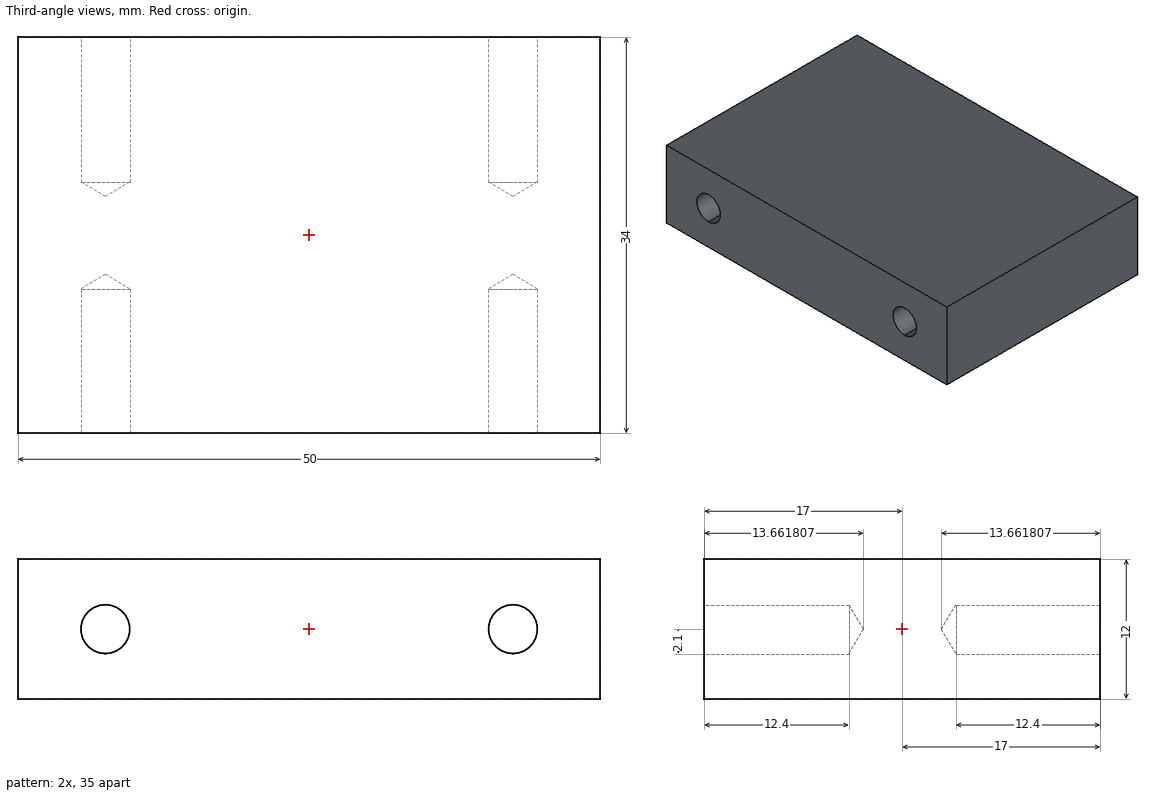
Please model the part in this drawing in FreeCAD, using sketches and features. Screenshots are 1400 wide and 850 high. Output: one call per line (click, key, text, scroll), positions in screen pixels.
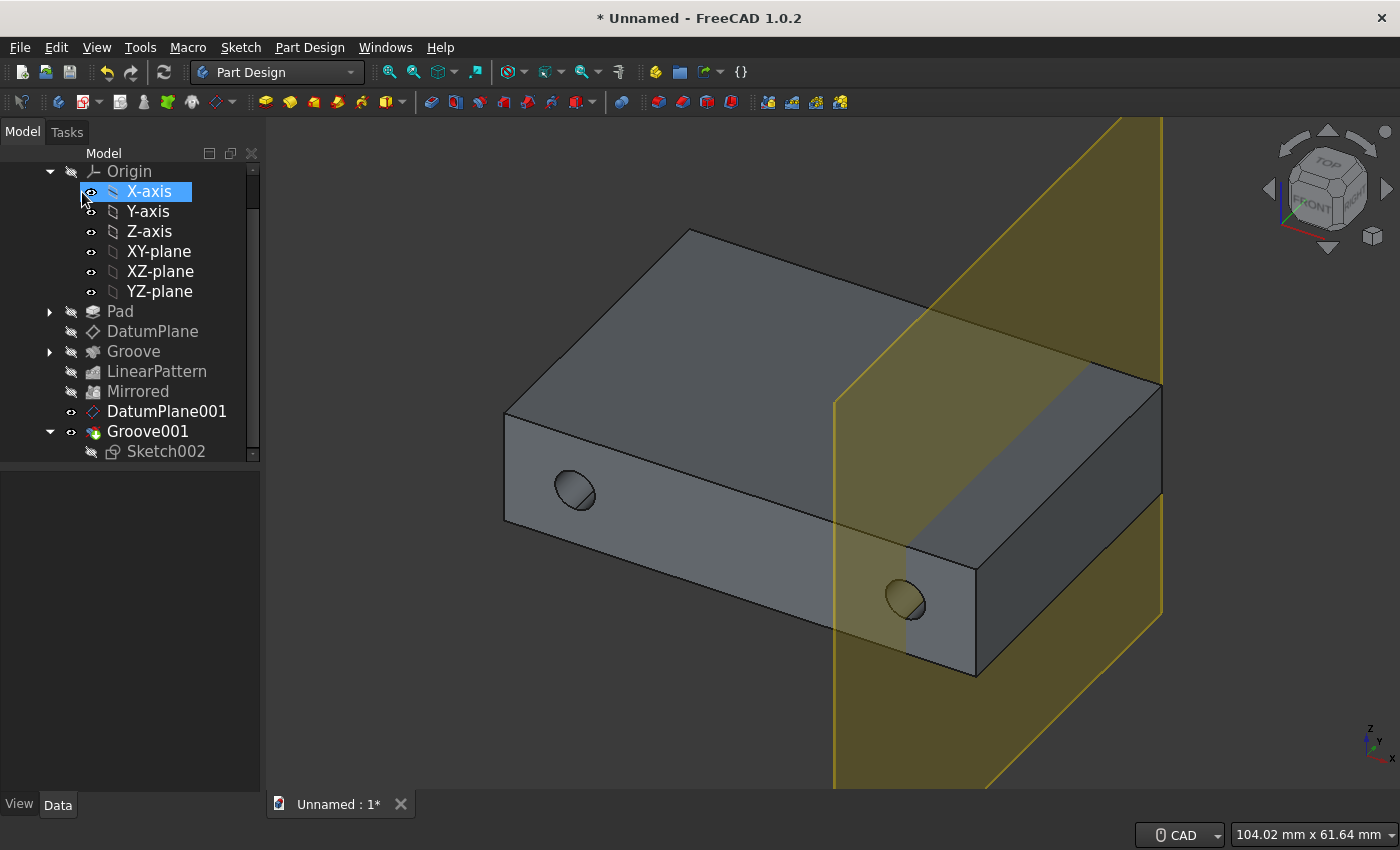
click(116, 412)
key(space)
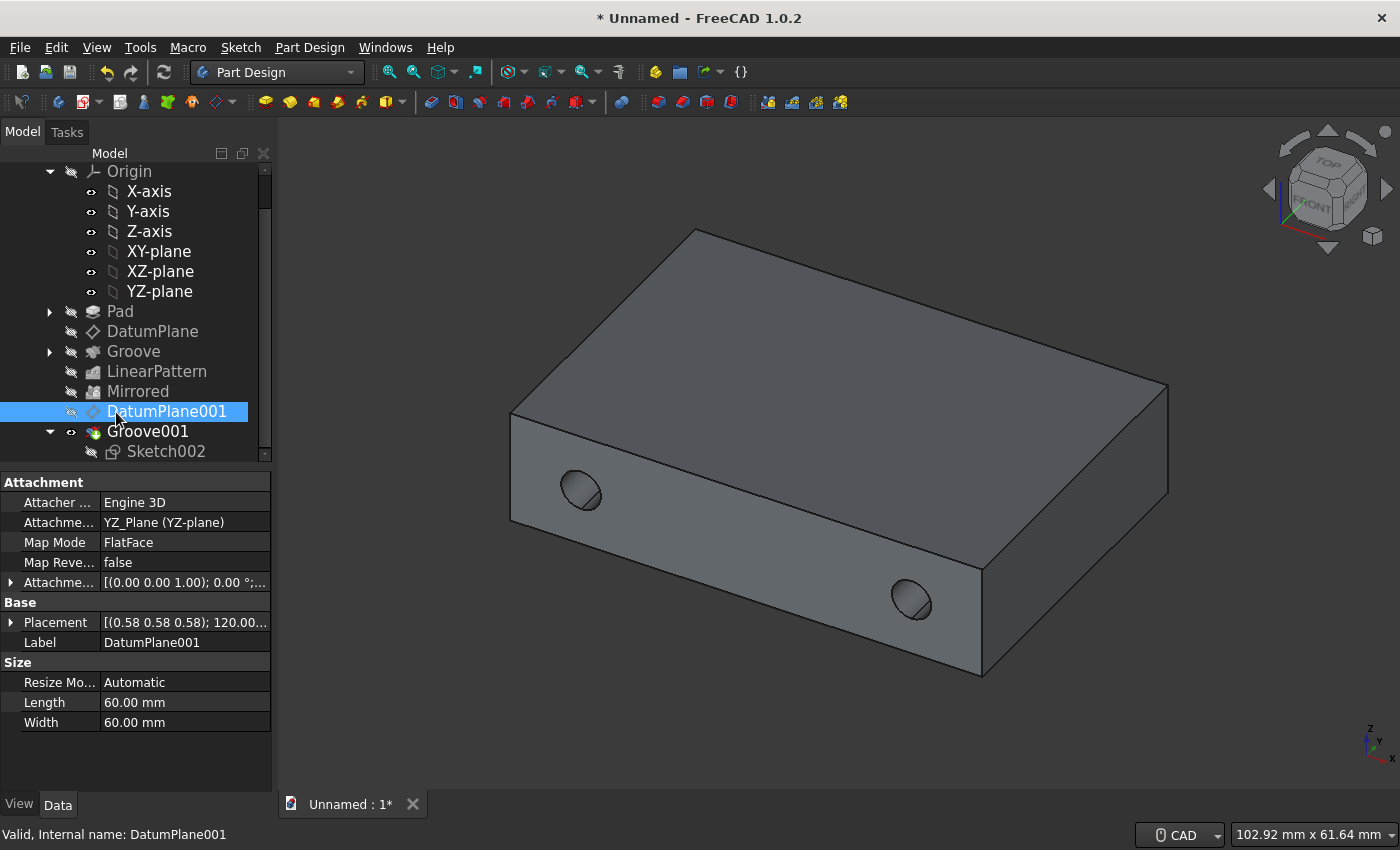
key(0)